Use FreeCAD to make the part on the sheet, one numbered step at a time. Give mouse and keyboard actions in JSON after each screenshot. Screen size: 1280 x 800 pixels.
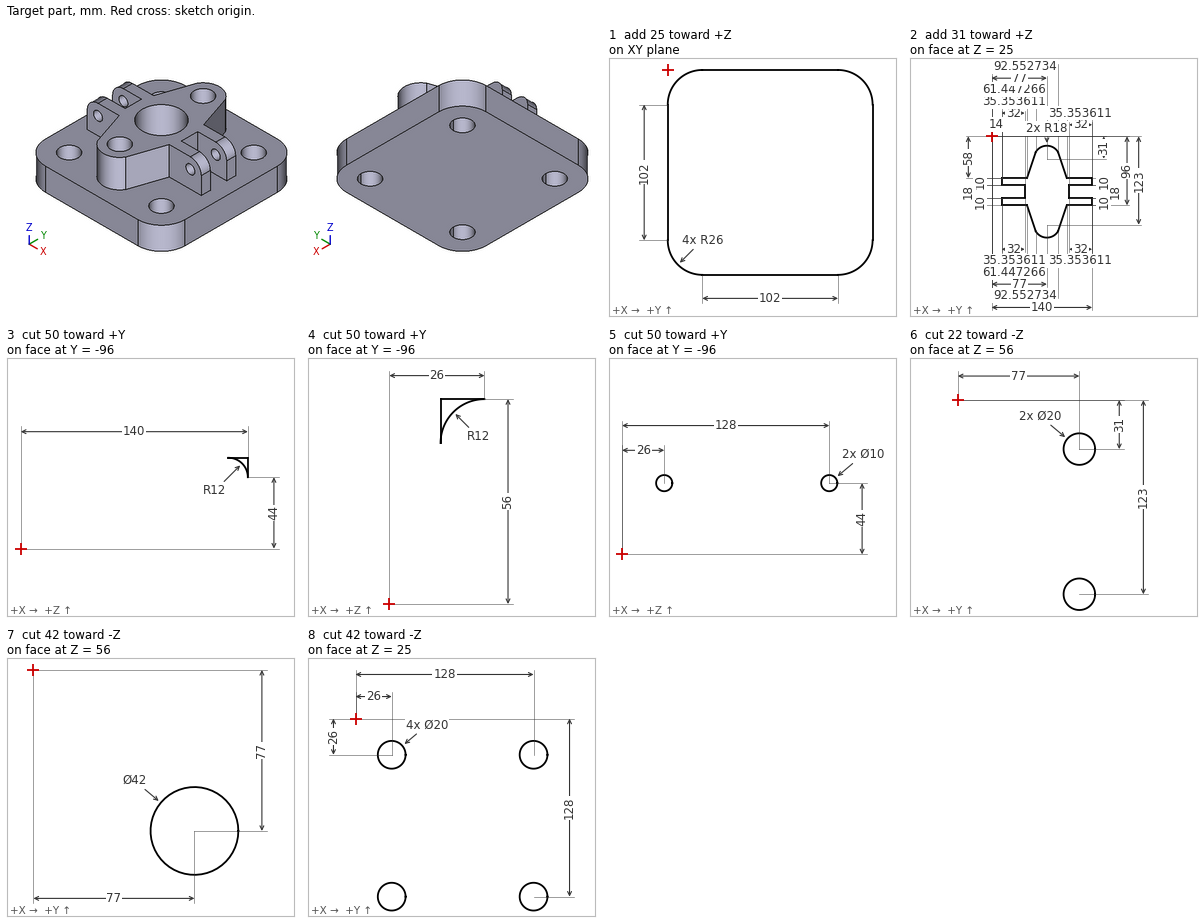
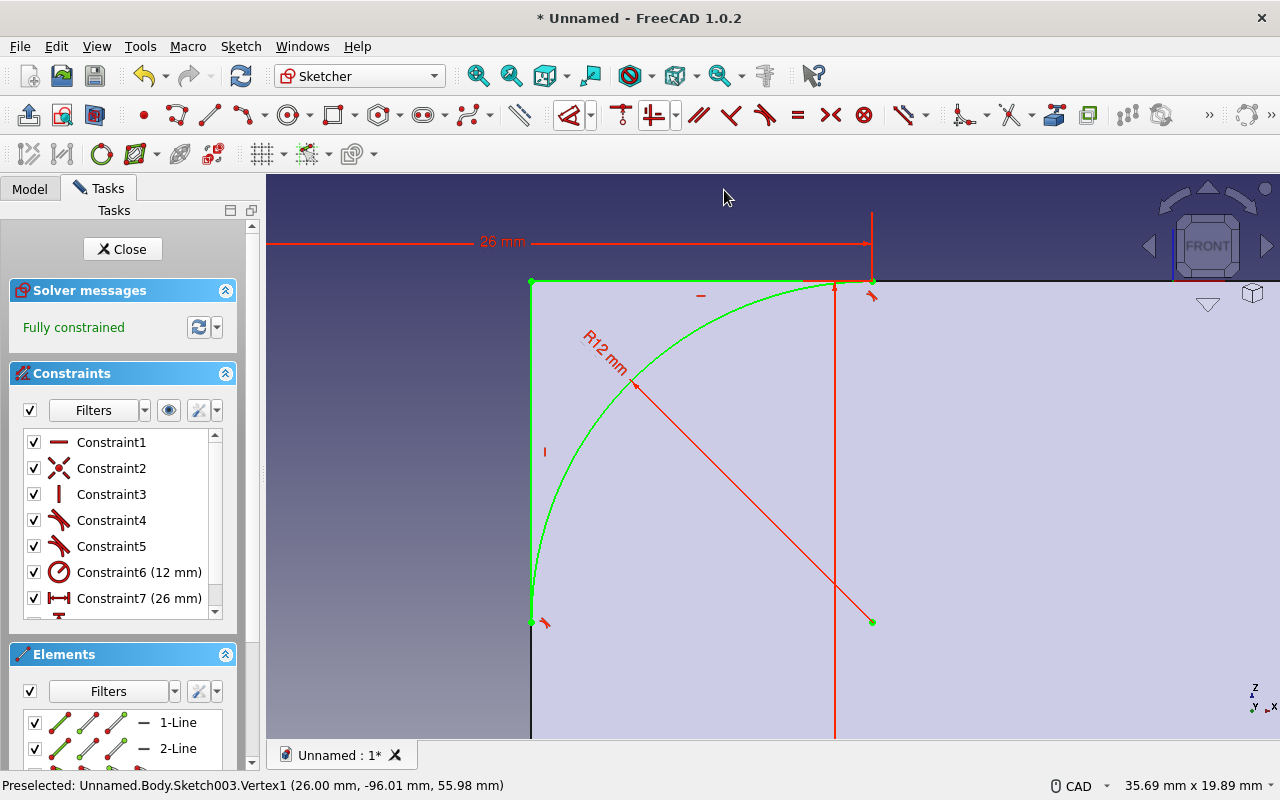
{"action": "left_click", "coordinate": [123, 249]}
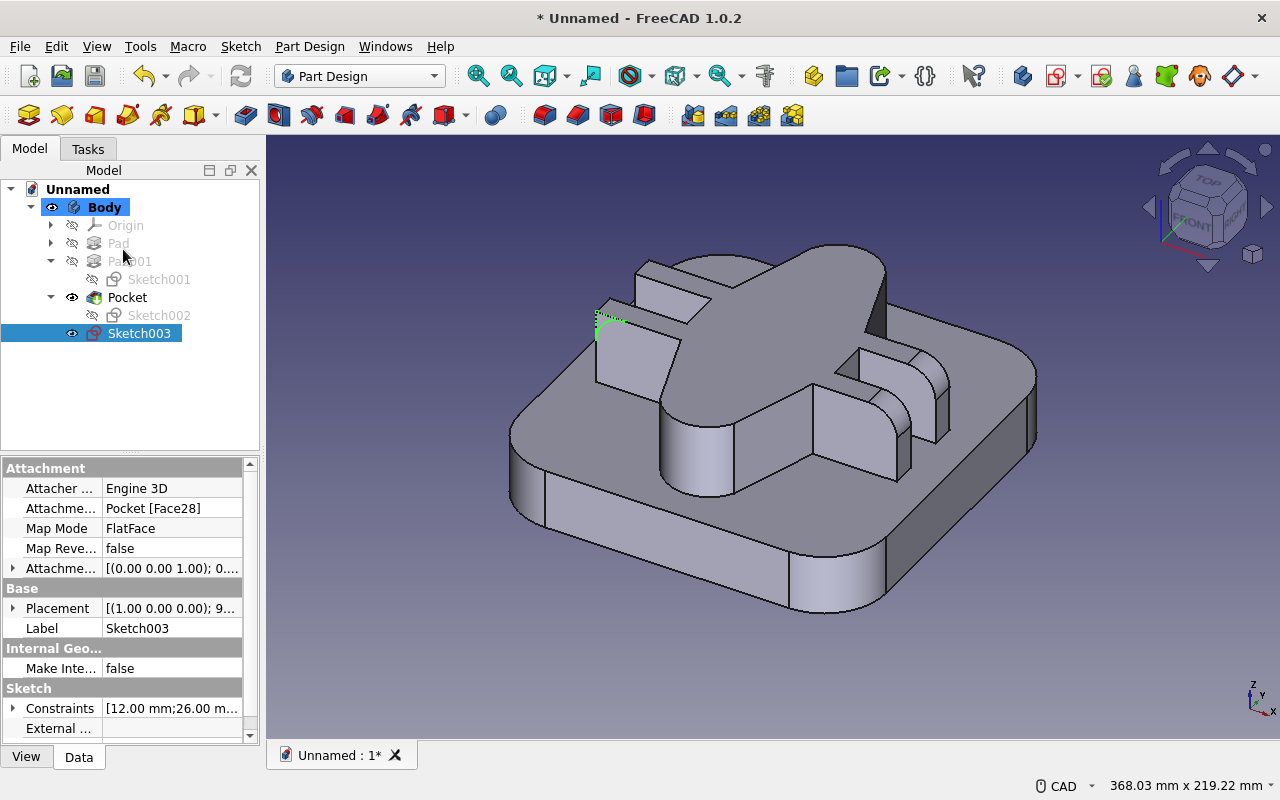
{"action": "left_click", "coordinate": [246, 116]}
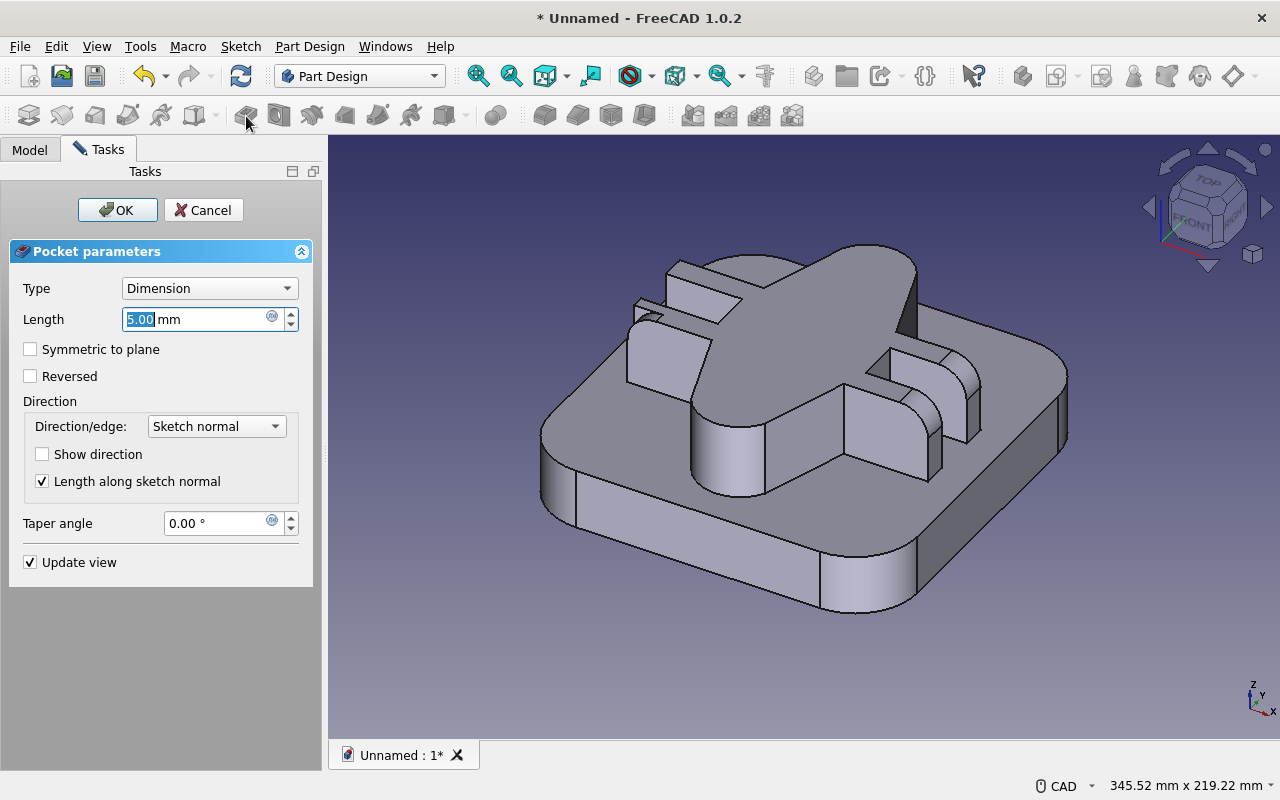
{"action": "type", "text": "50"}
{"action": "key", "text": "Tab"}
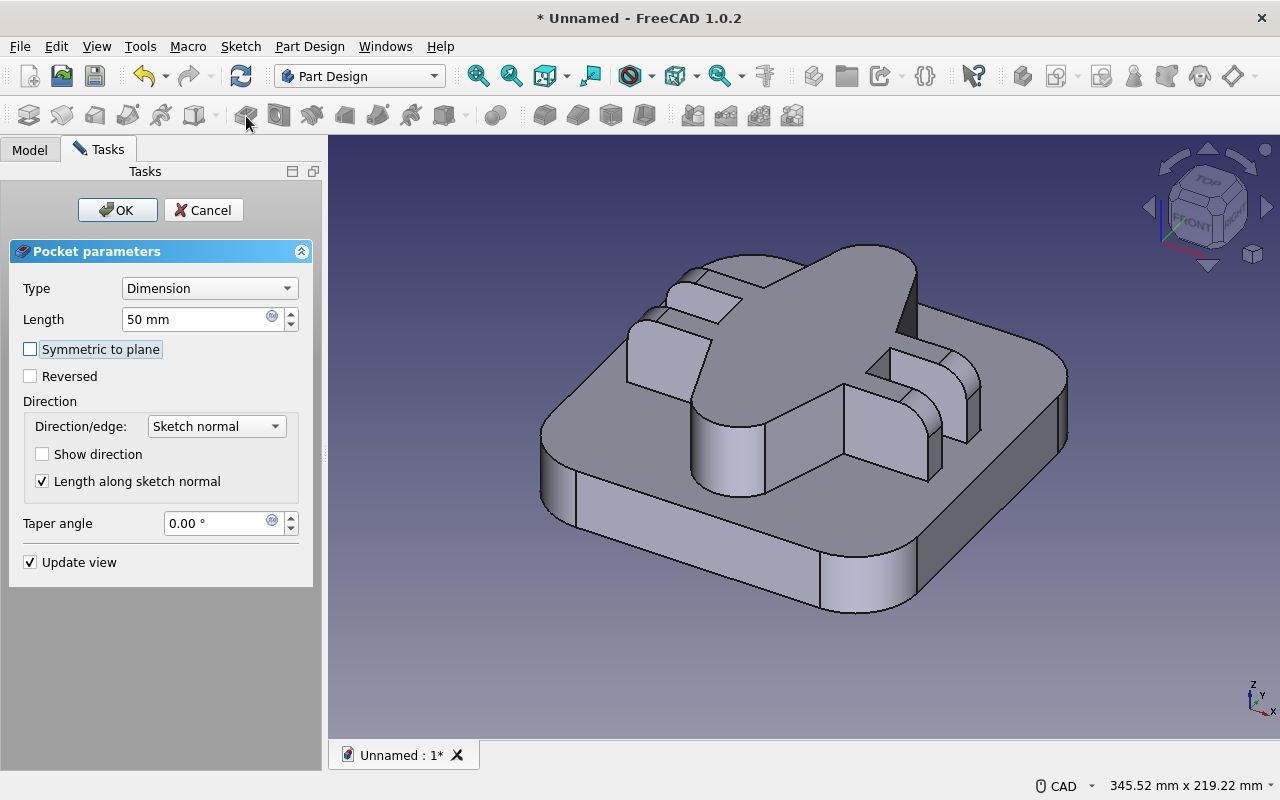
{"action": "left_click", "coordinate": [118, 210]}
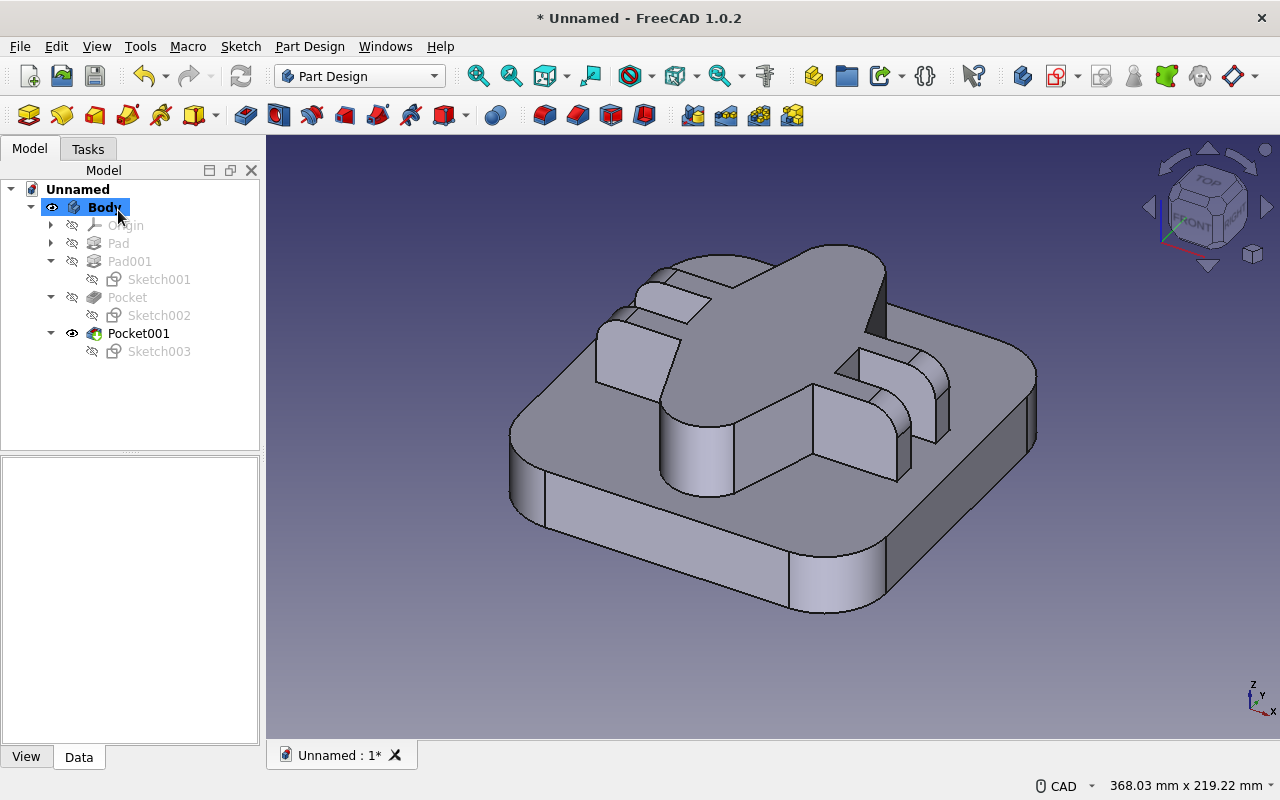
{"action": "left_click", "coordinate": [639, 360]}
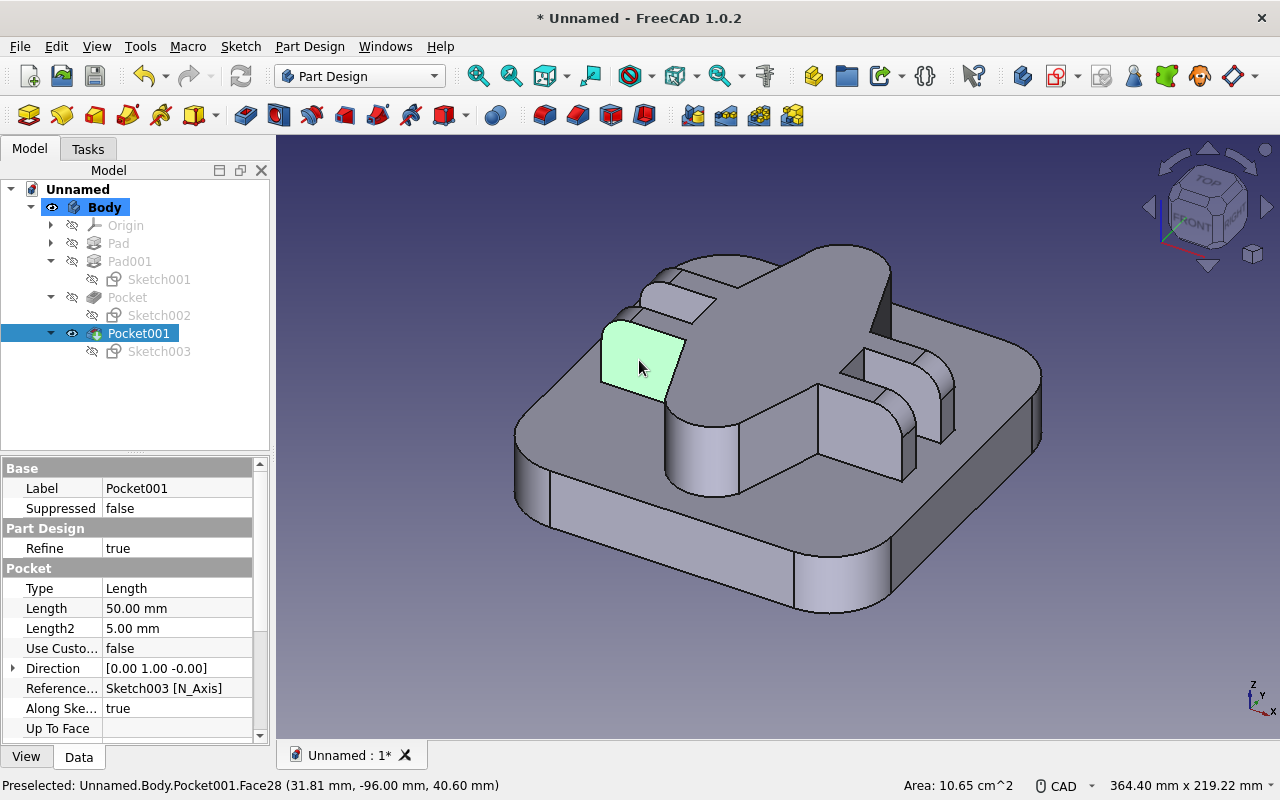
{"action": "left_click", "coordinate": [1056, 76]}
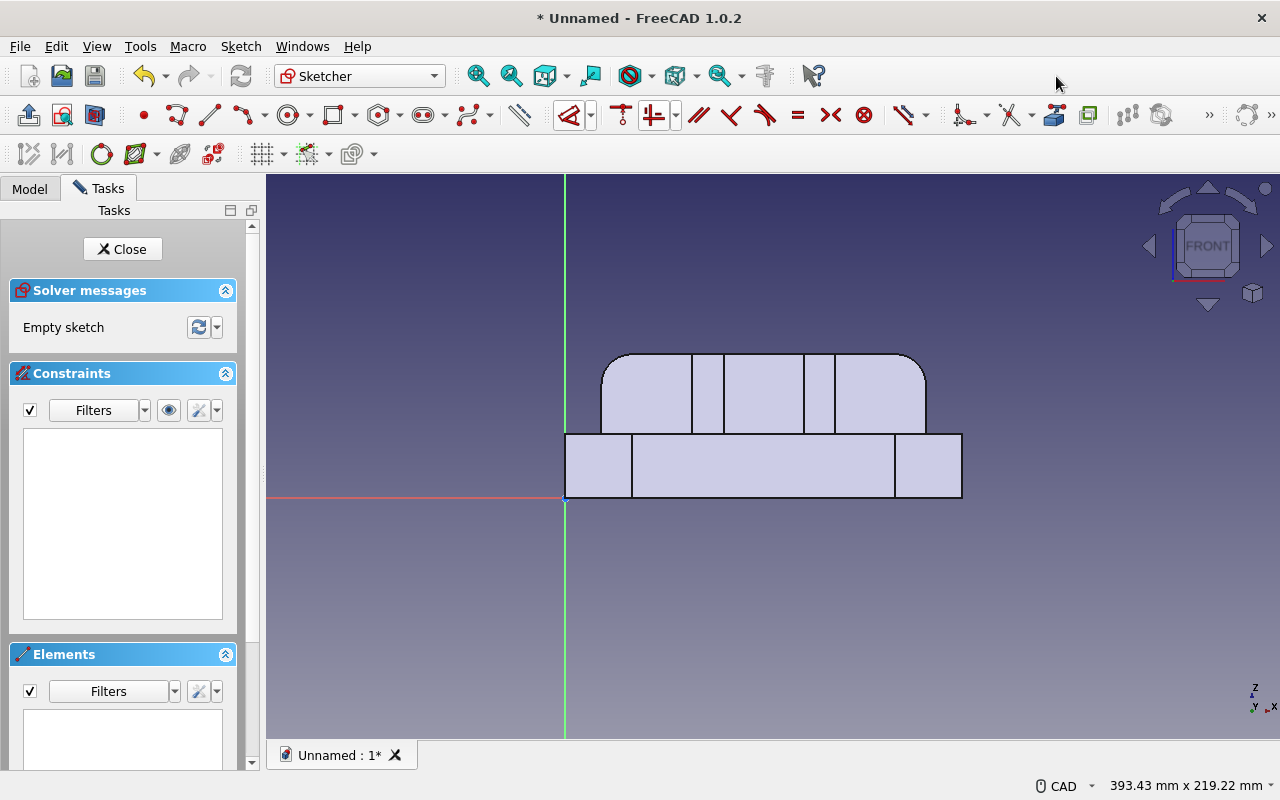
{"action": "scroll", "coordinate": [776, 409], "scroll_direction": "up", "scroll_amount": 3}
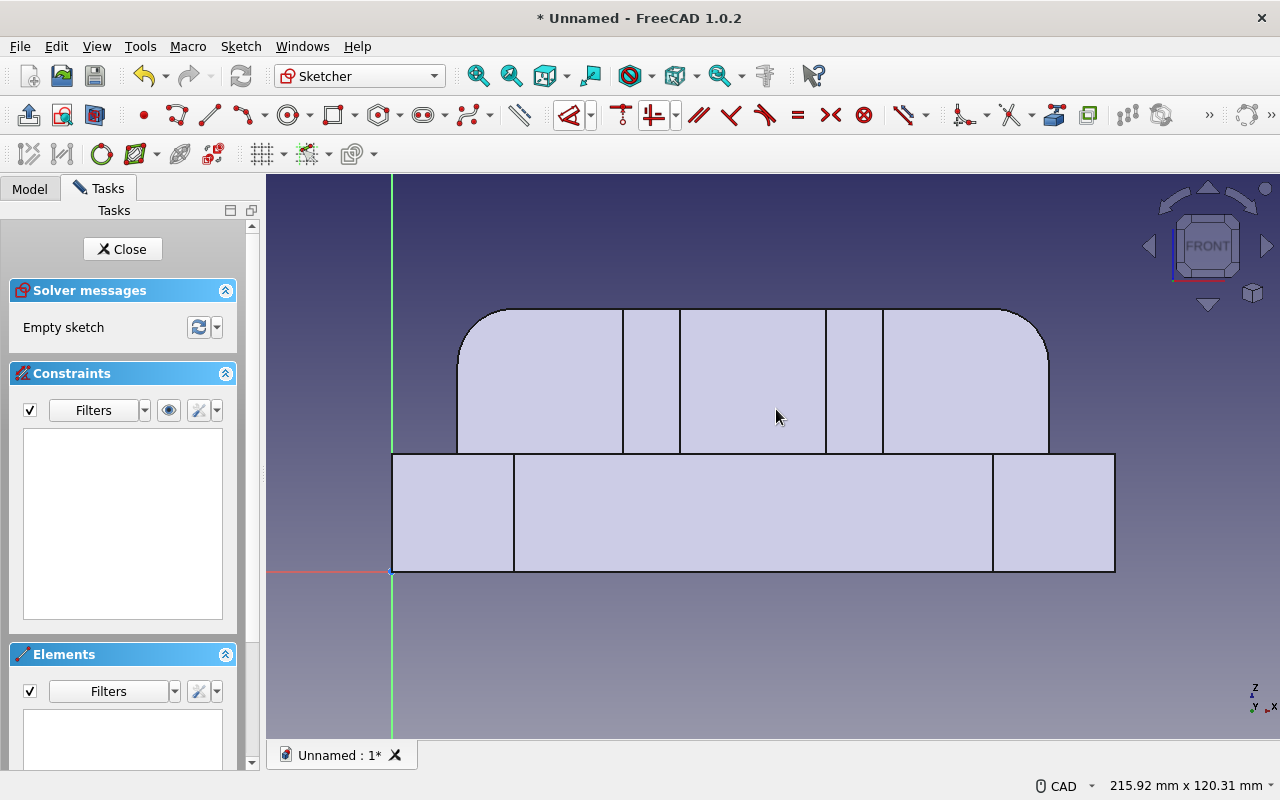
{"action": "left_click", "coordinate": [288, 116]}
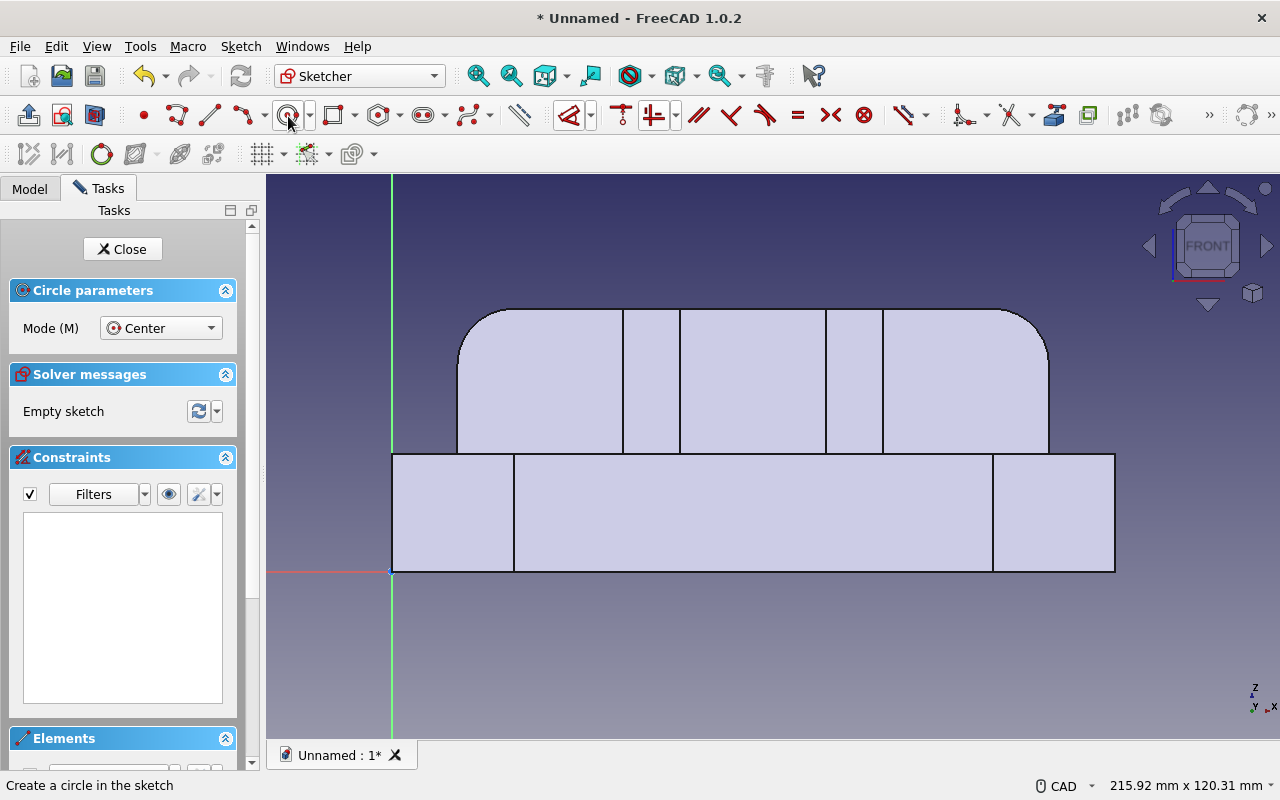
{"action": "left_click", "coordinate": [993, 365]}
{"action": "left_click", "coordinate": [1009, 348]}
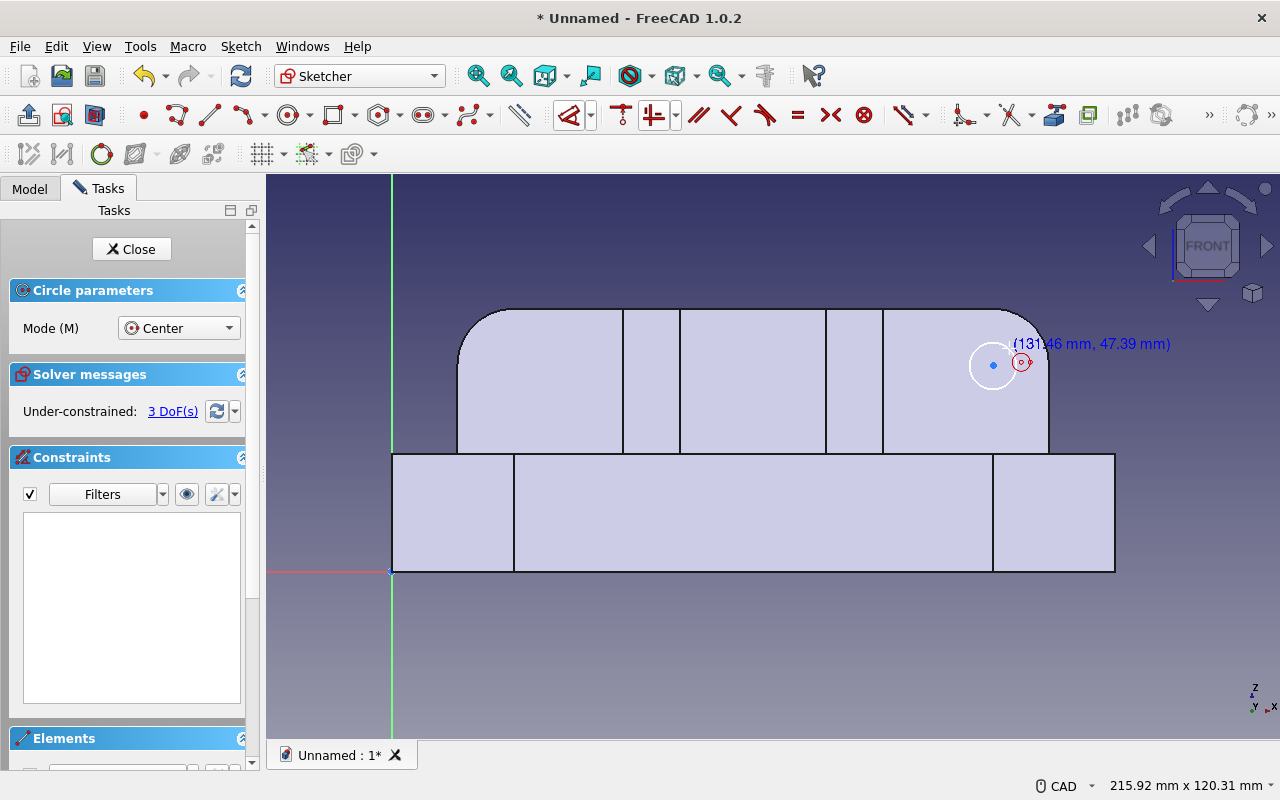
{"action": "left_click", "coordinate": [514, 365]}
{"action": "left_click", "coordinate": [530, 348]}
{"action": "key", "text": "Escape"}